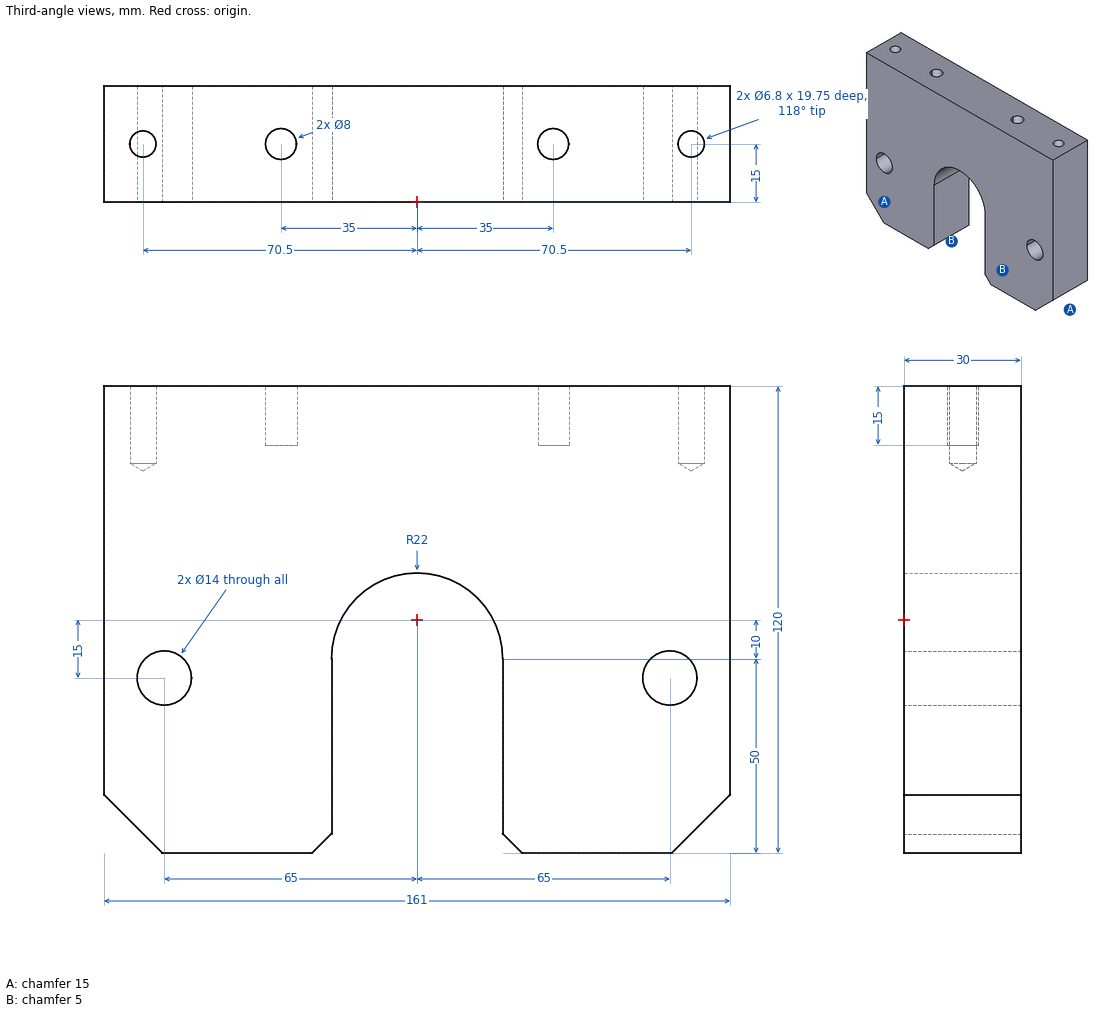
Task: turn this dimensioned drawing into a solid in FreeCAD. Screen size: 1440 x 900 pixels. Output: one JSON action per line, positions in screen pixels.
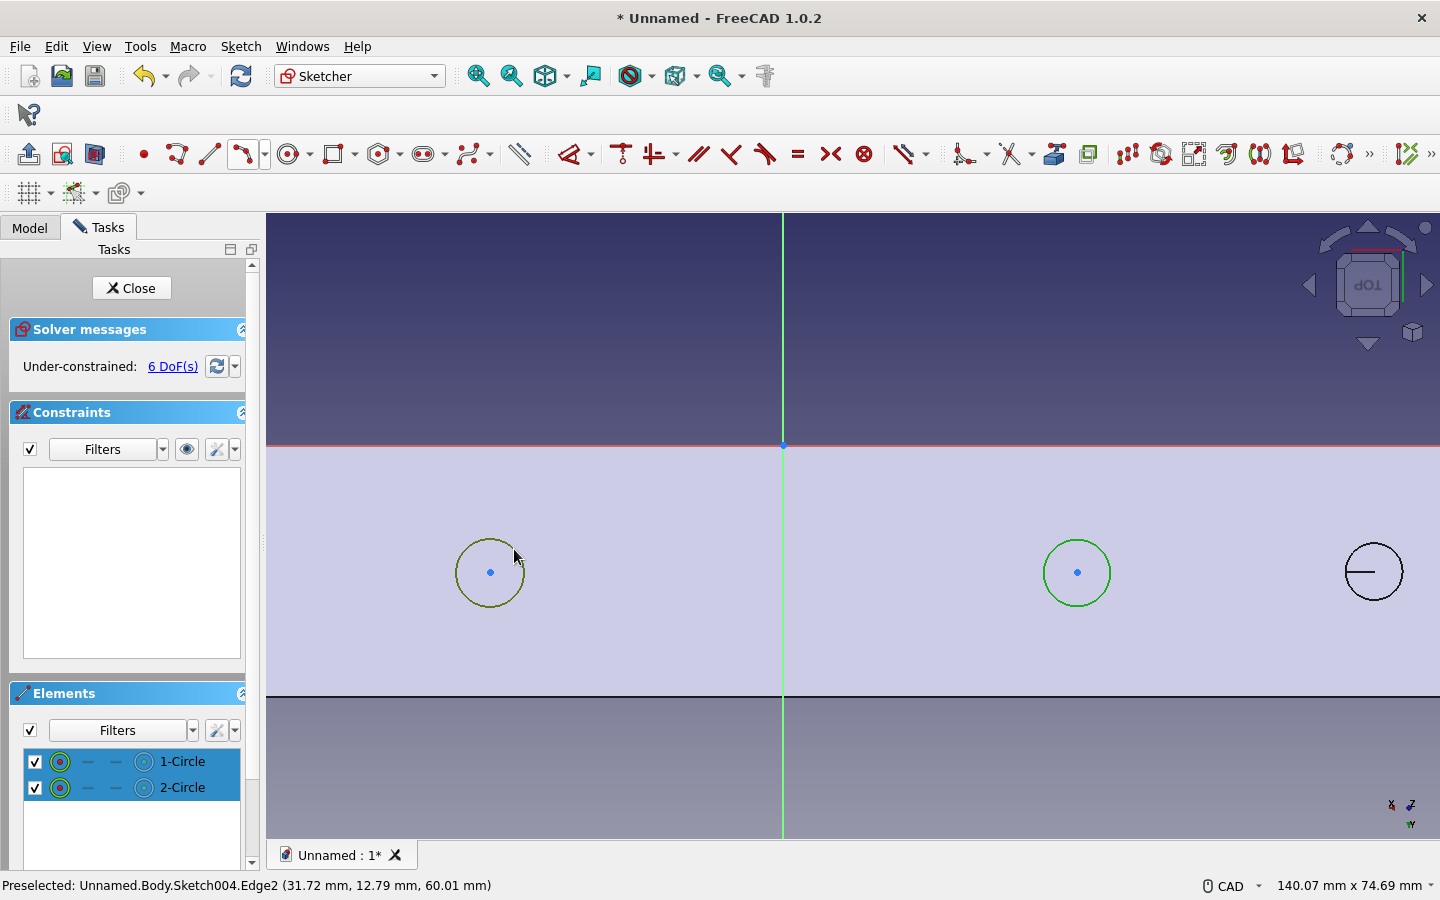
{"action": "key", "text": "e"}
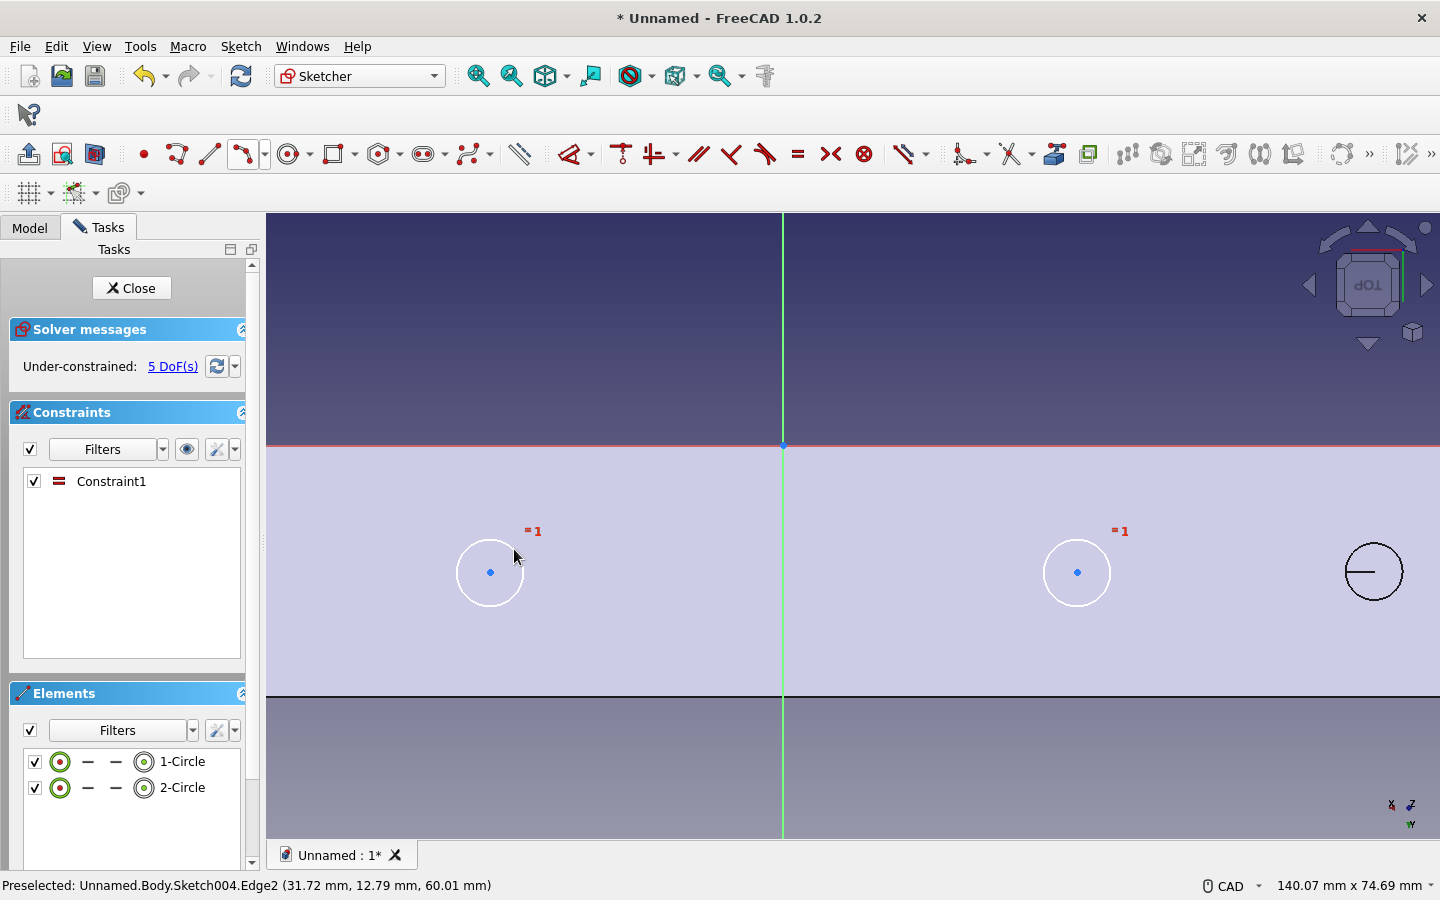
{"action": "left_click", "coordinate": [1077, 573]}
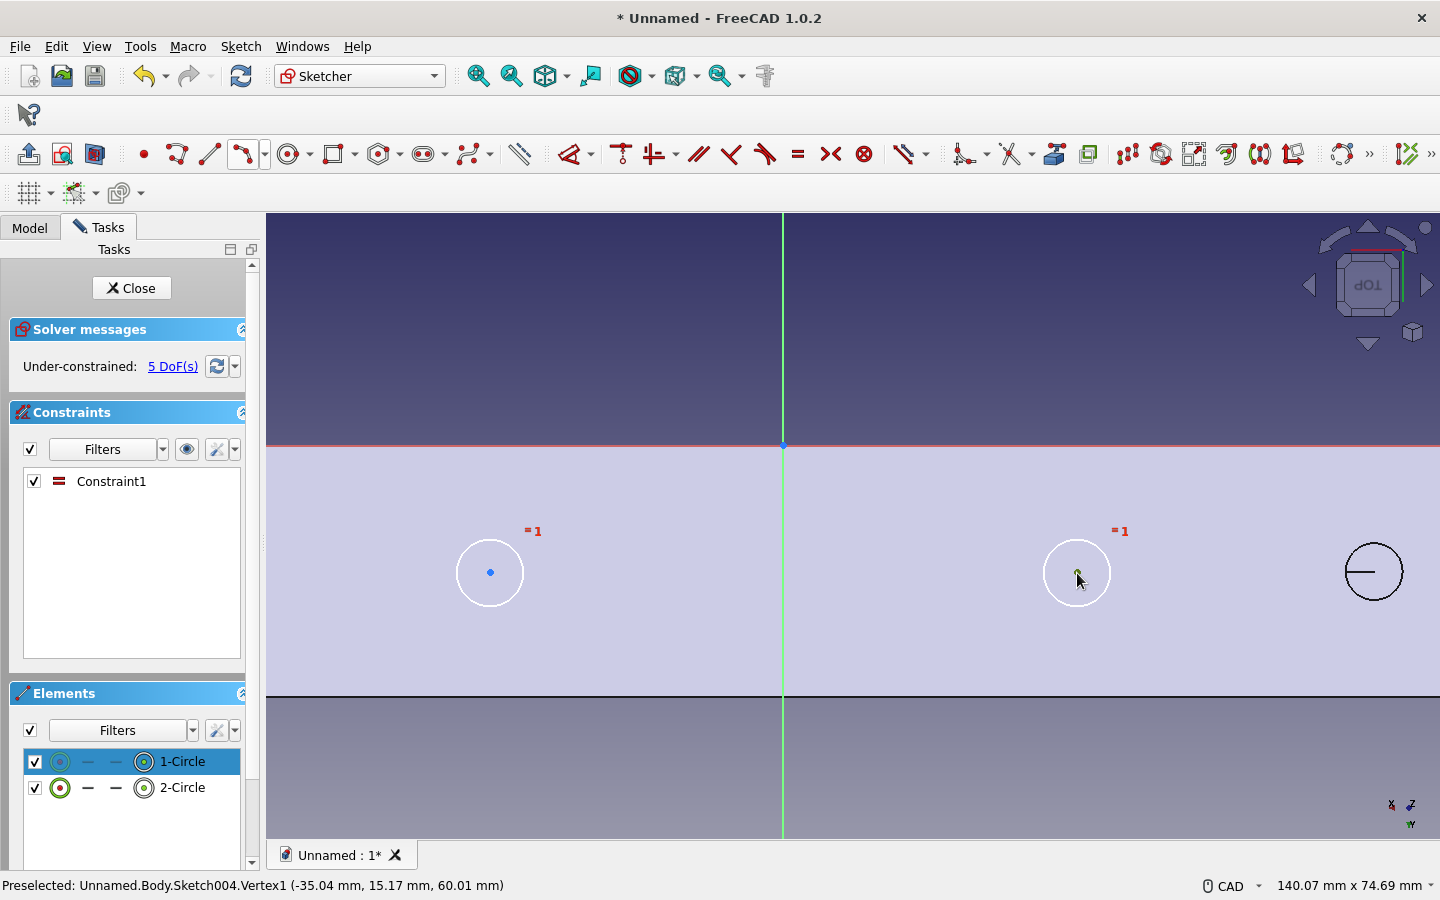
{"action": "left_click", "coordinate": [490, 573]}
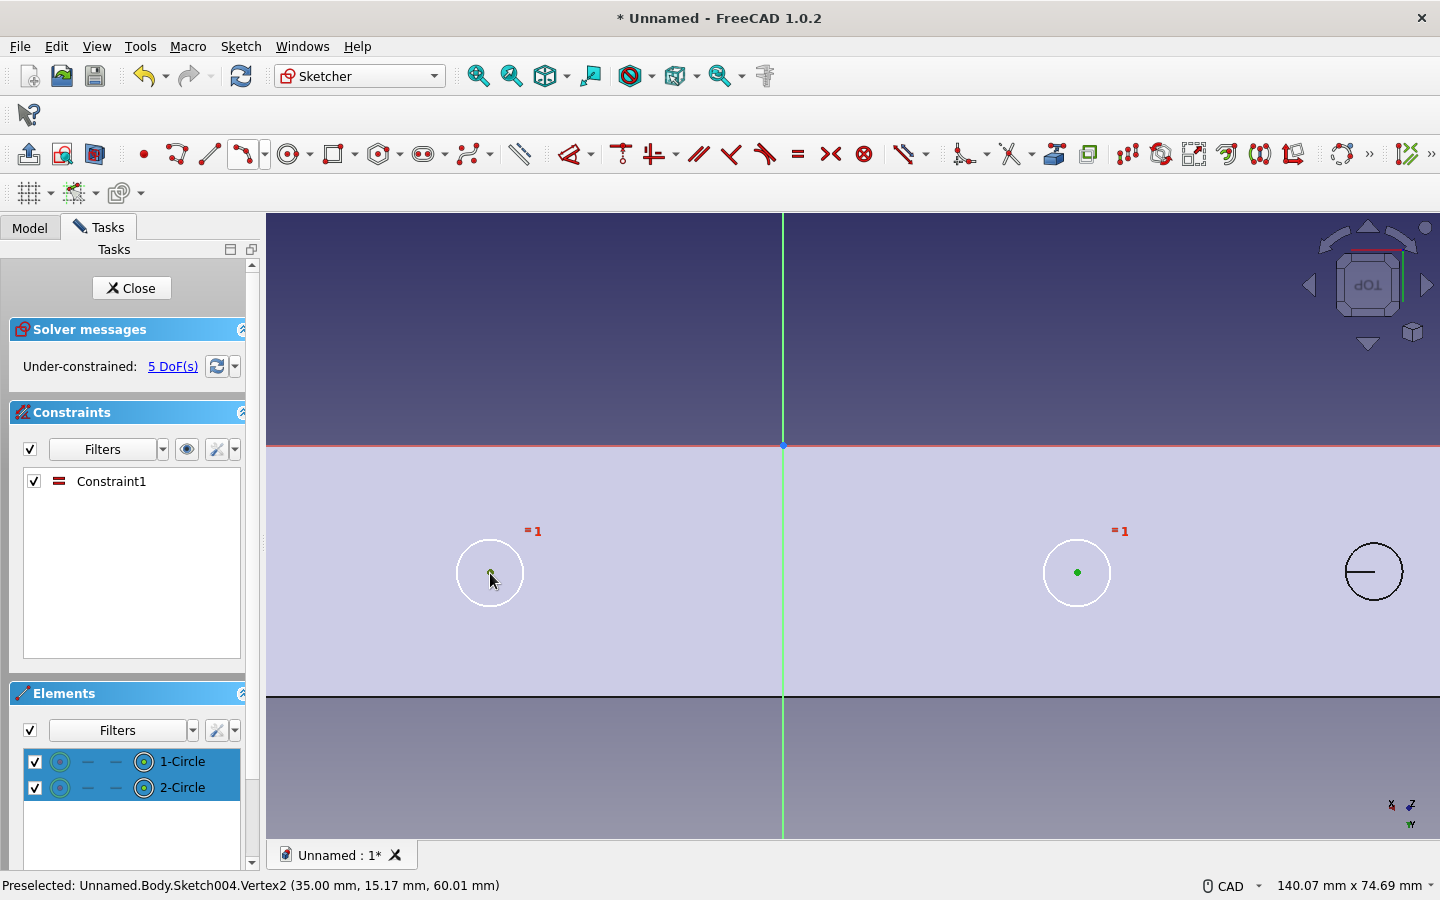
{"action": "key", "text": "h"}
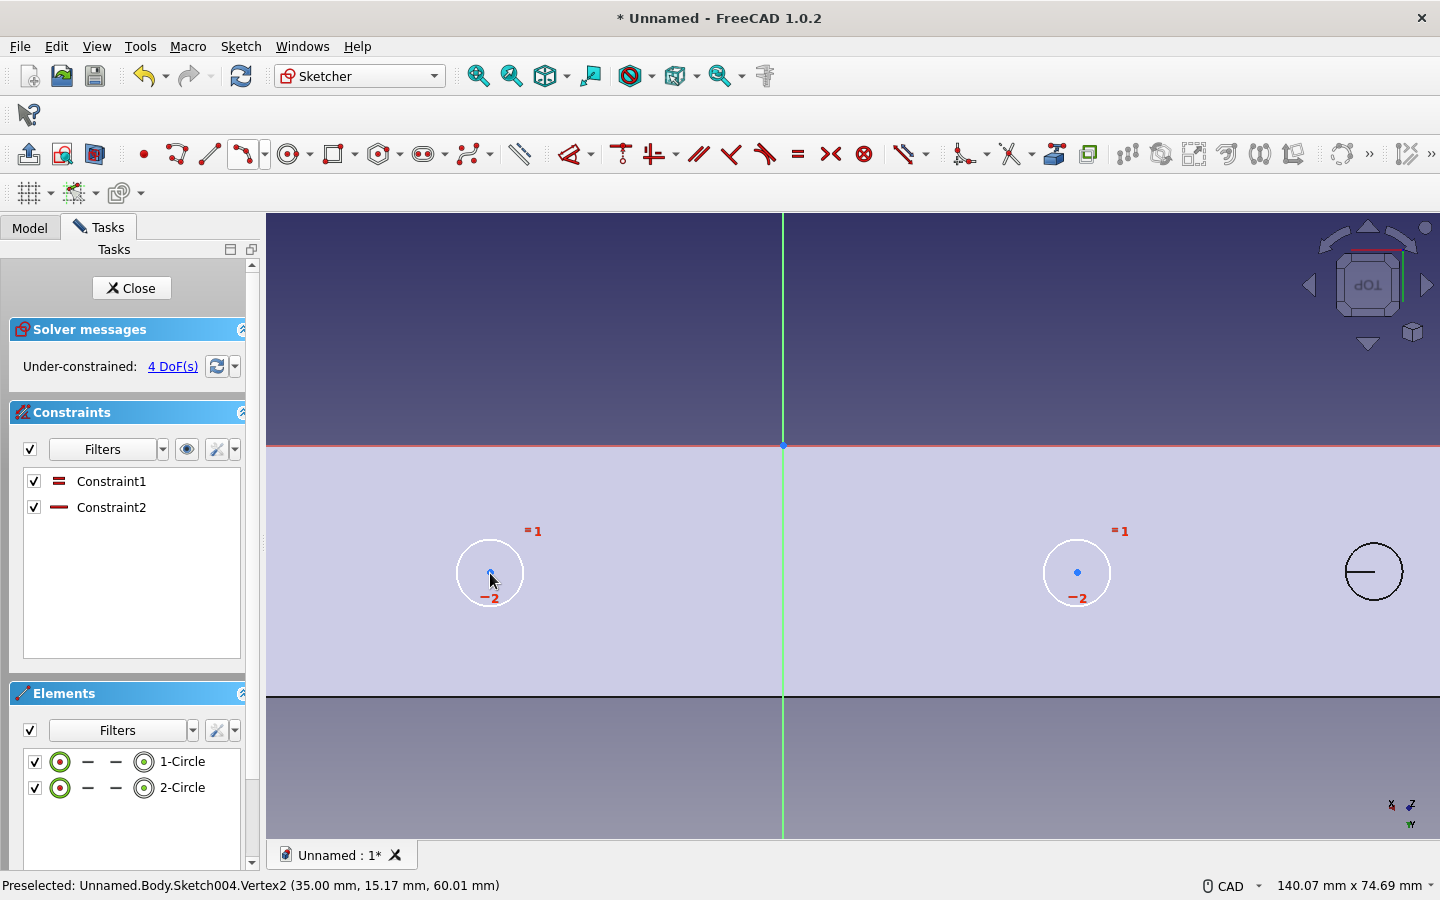
{"action": "key", "text": "d"}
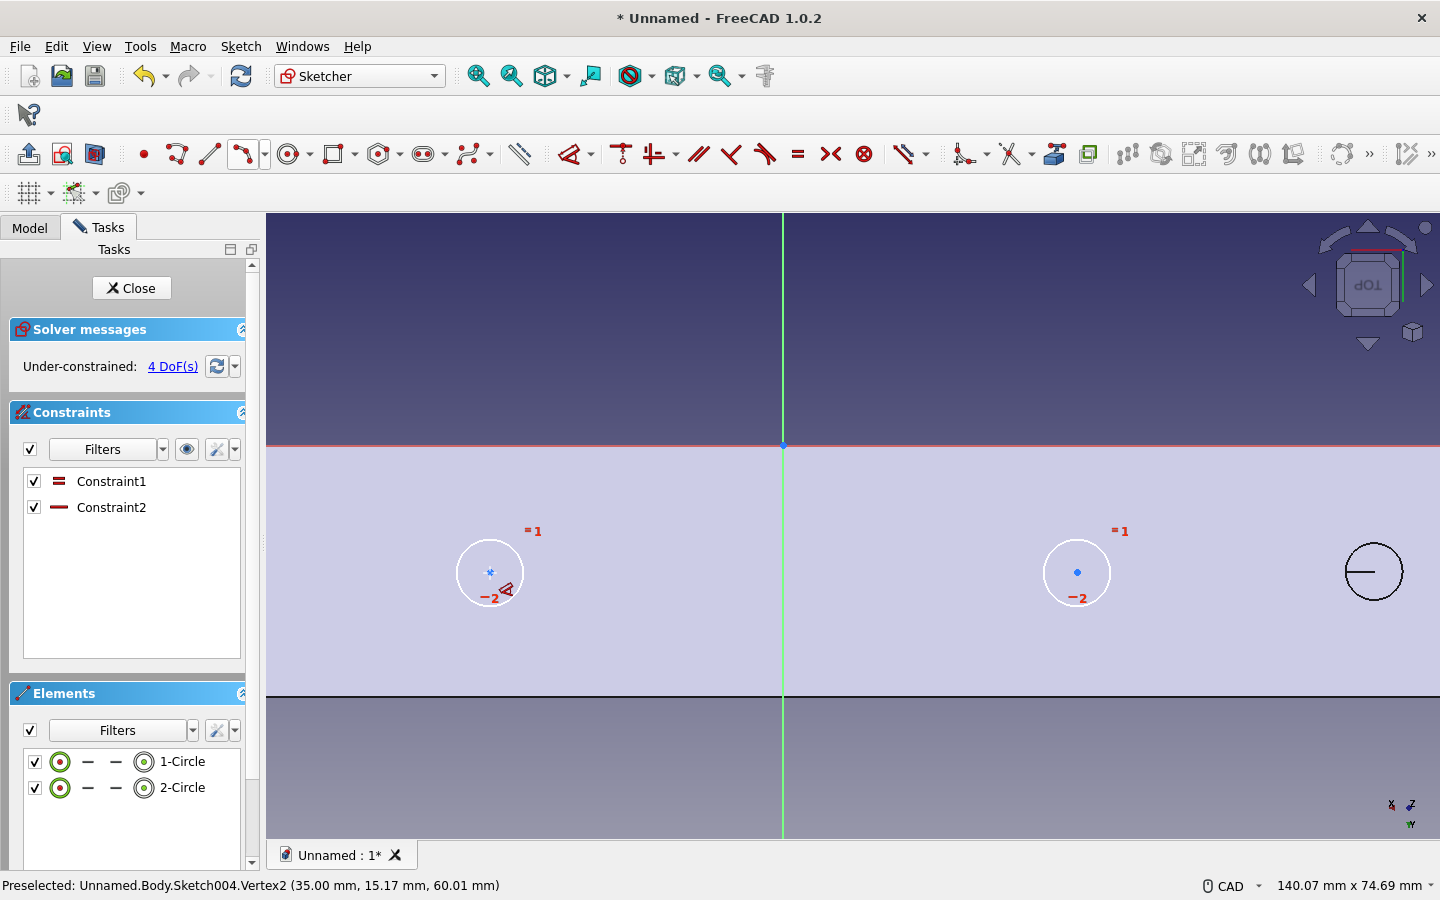
{"action": "left_click", "coordinate": [1100, 549]}
{"action": "left_click", "coordinate": [1122, 526]}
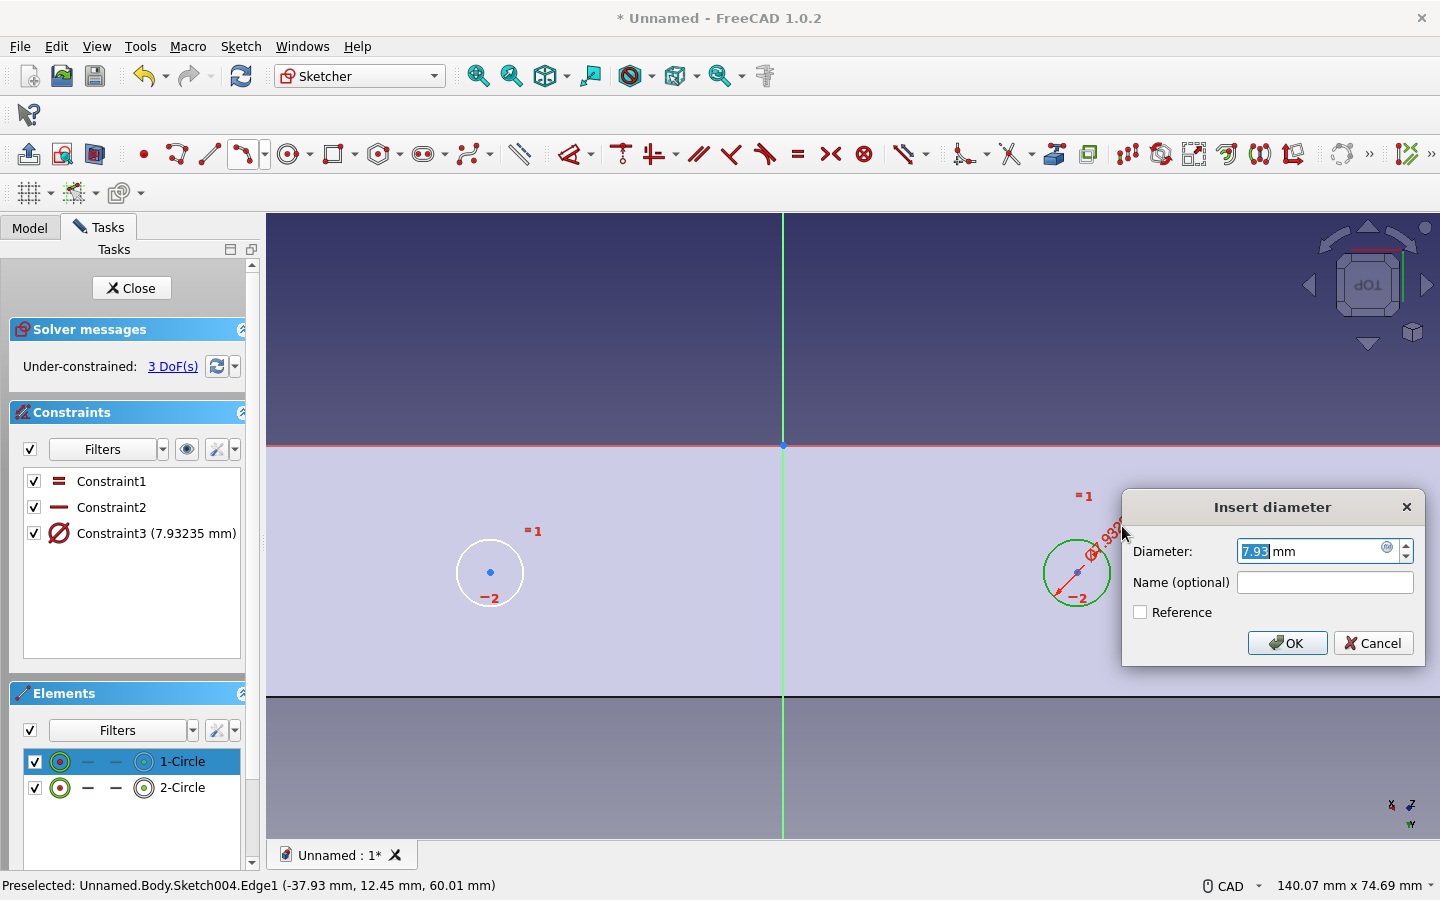
{"action": "type", "text": "8"}
{"action": "key", "text": "Return"}